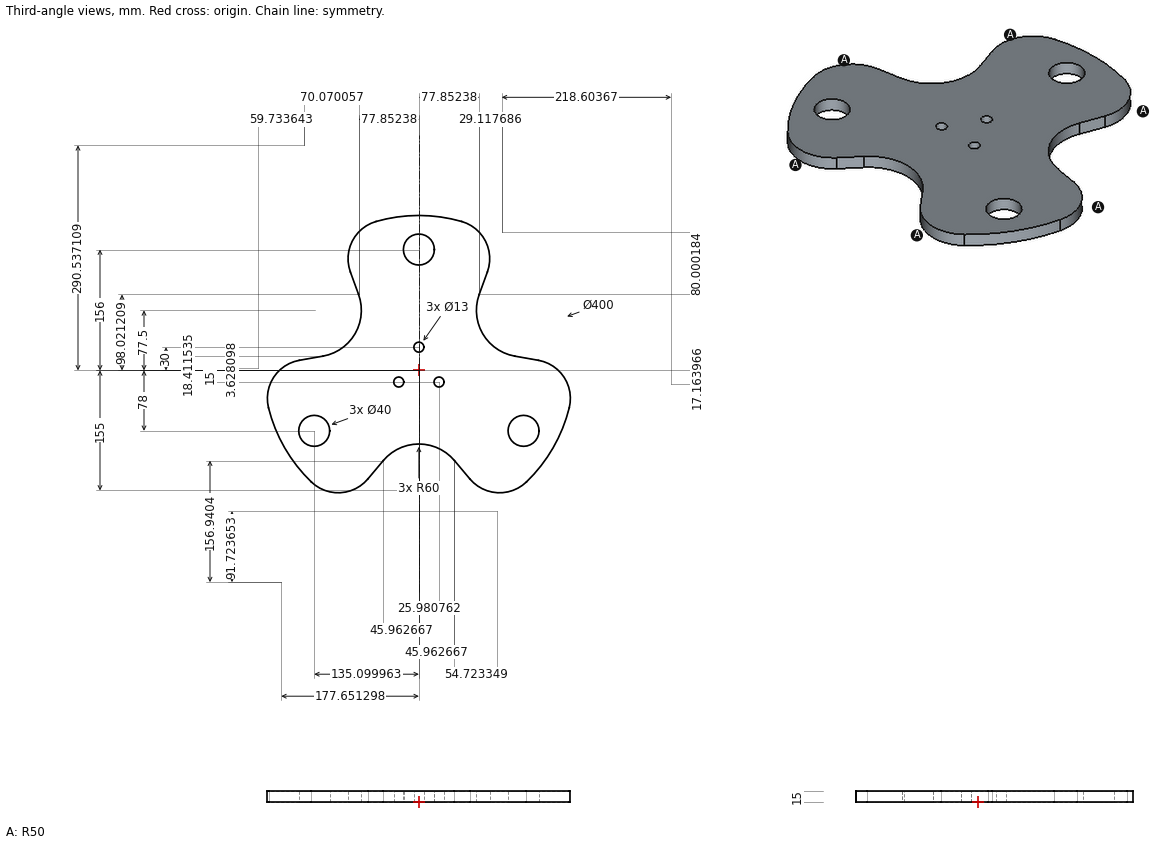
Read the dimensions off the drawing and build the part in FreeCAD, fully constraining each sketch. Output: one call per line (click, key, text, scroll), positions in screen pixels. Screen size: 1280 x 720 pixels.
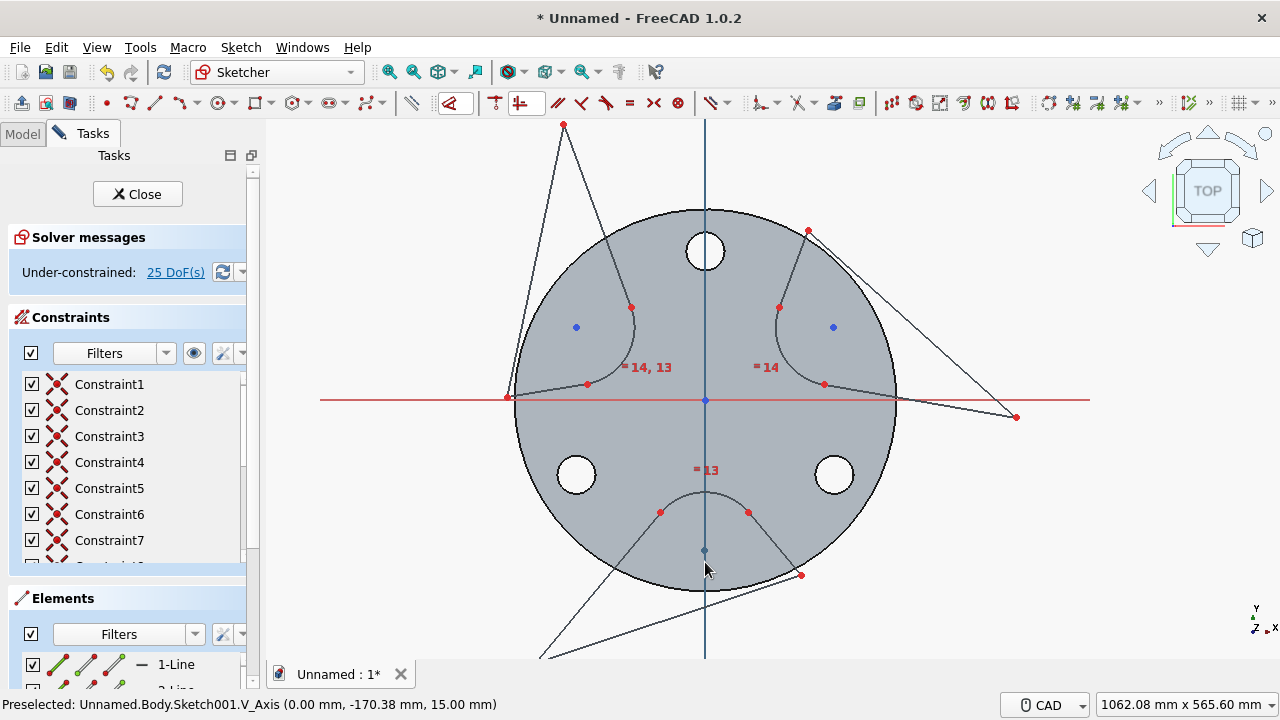
click(496, 104)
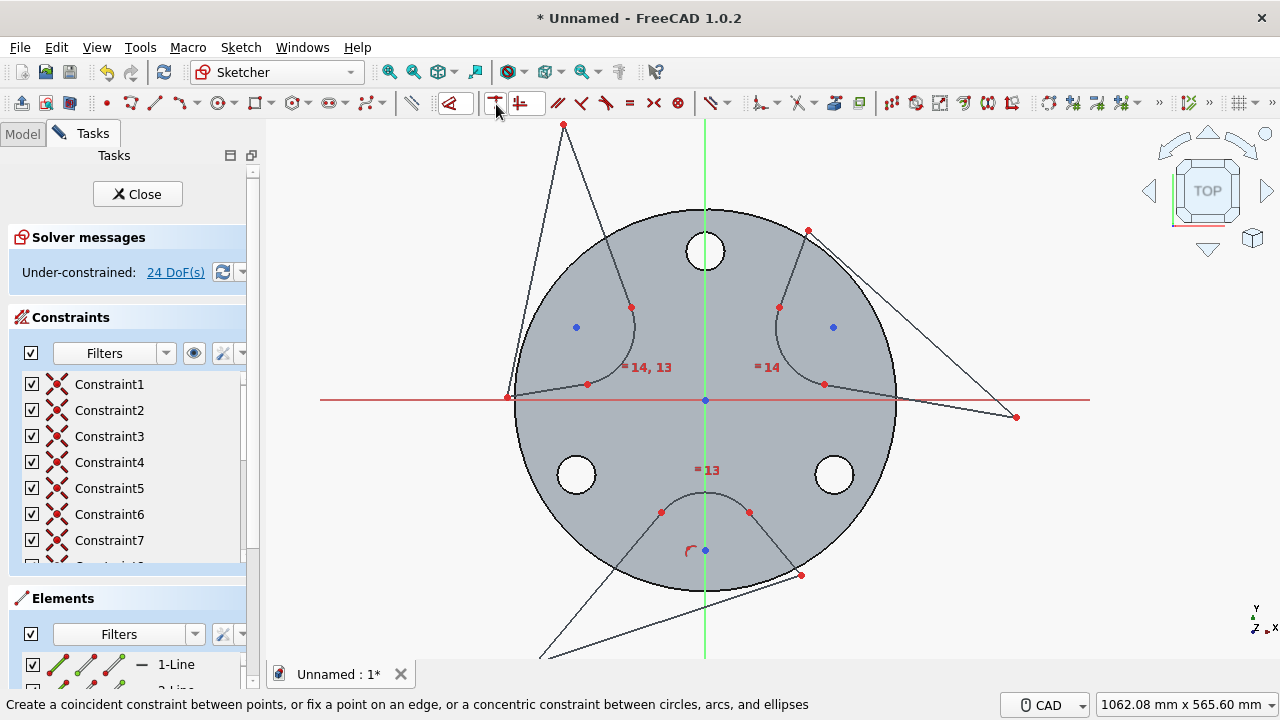
click(577, 327)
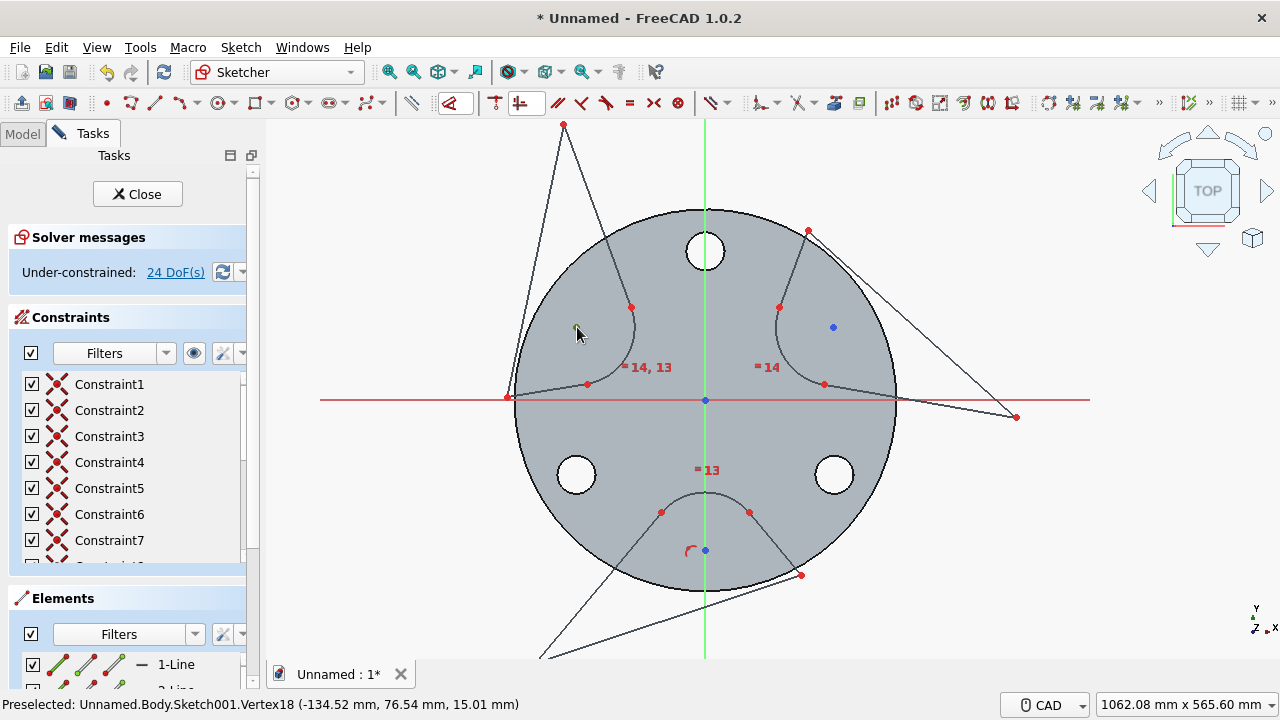
click(834, 328)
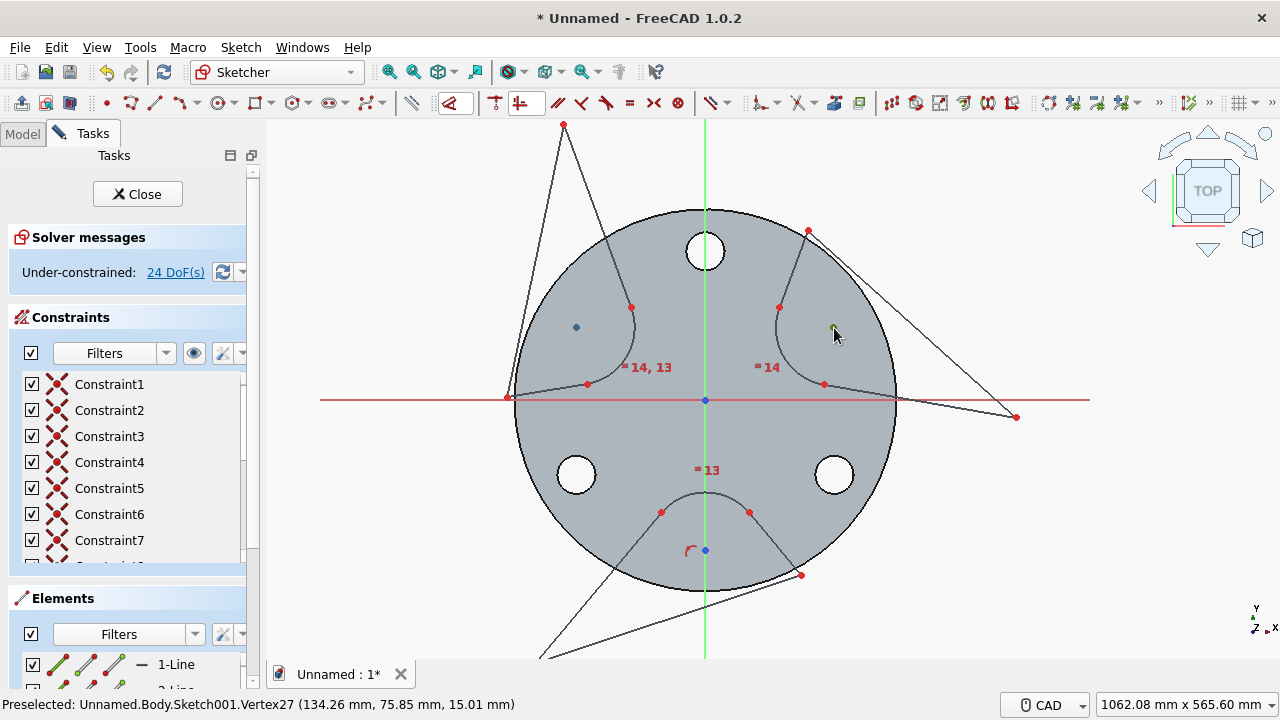
click(705, 562)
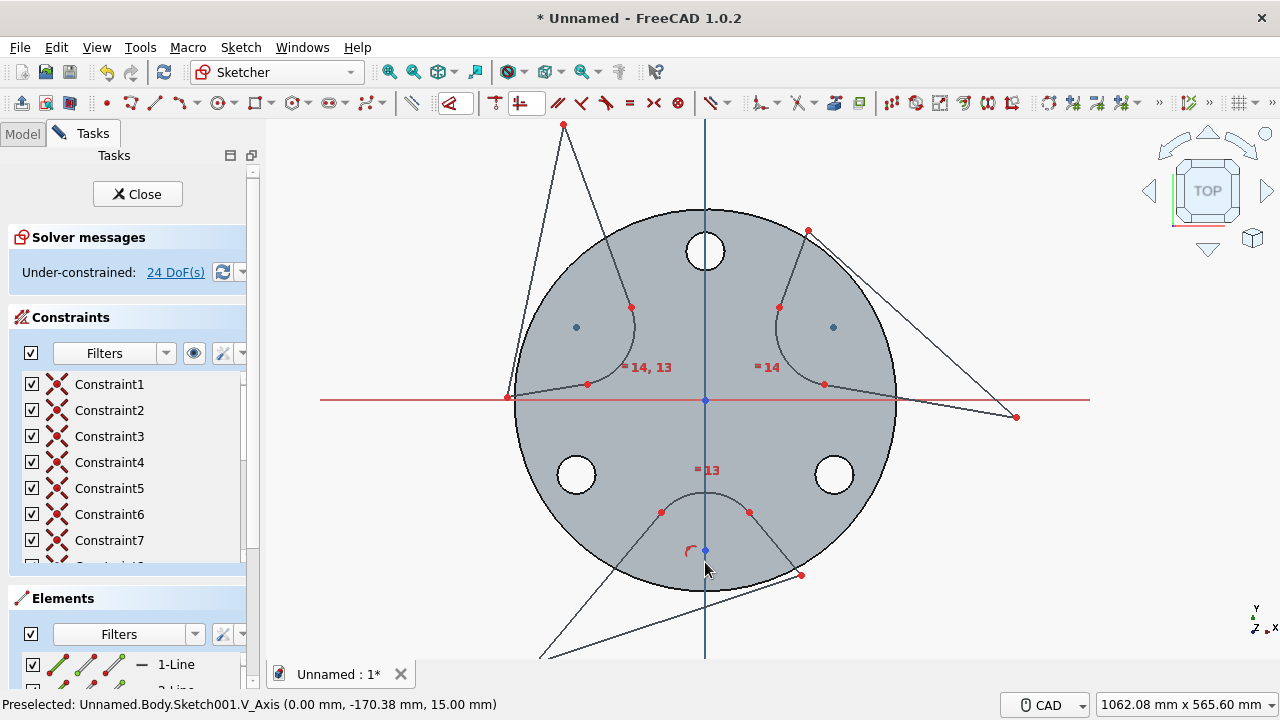
click(654, 104)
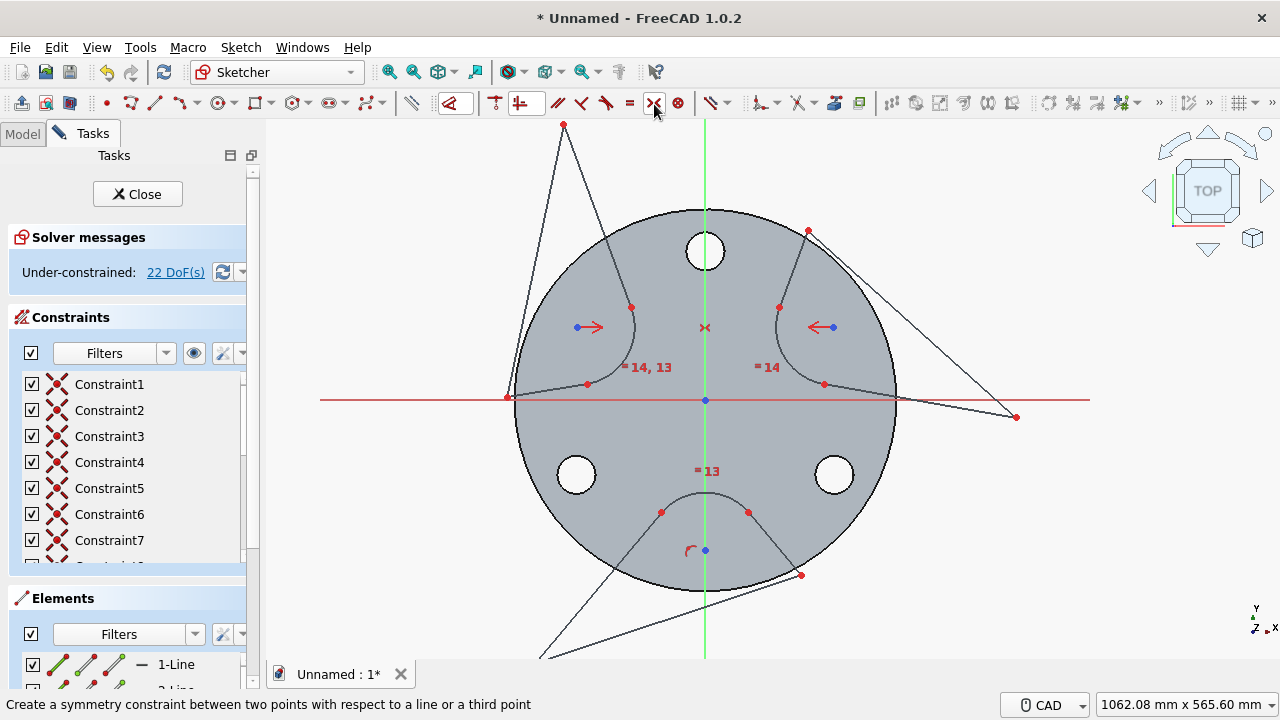
click(725, 496)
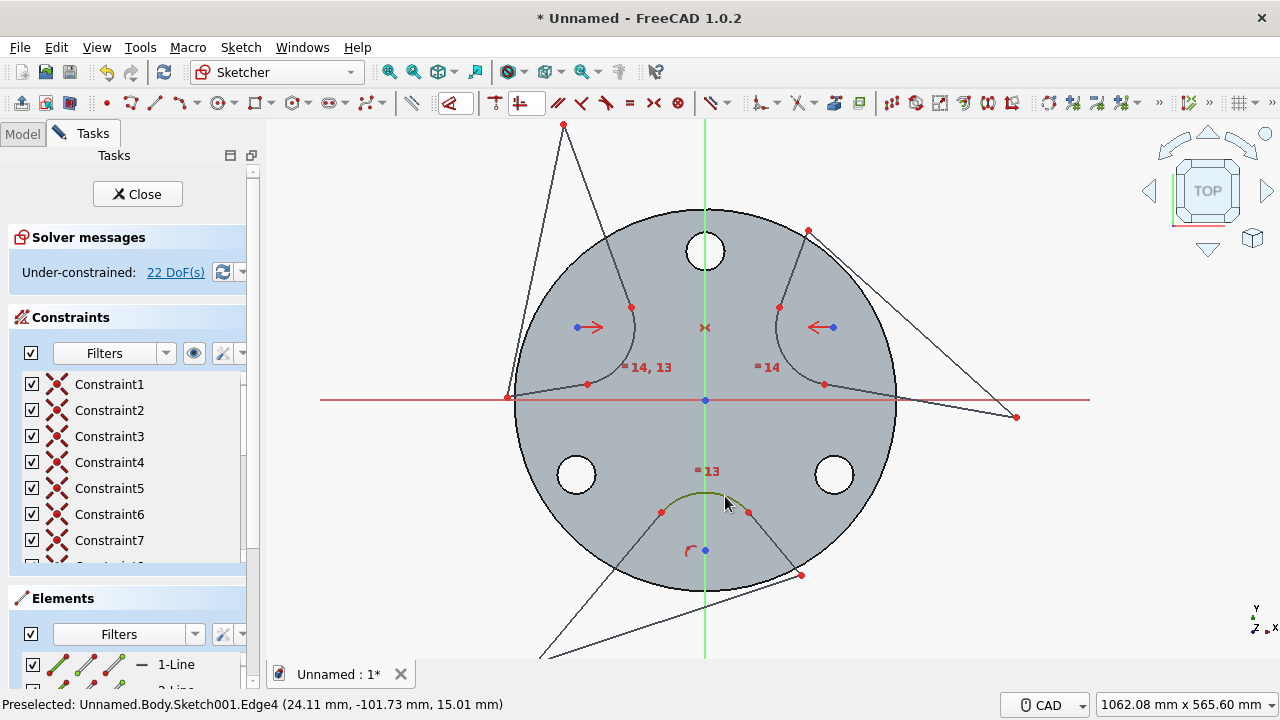
click(468, 104)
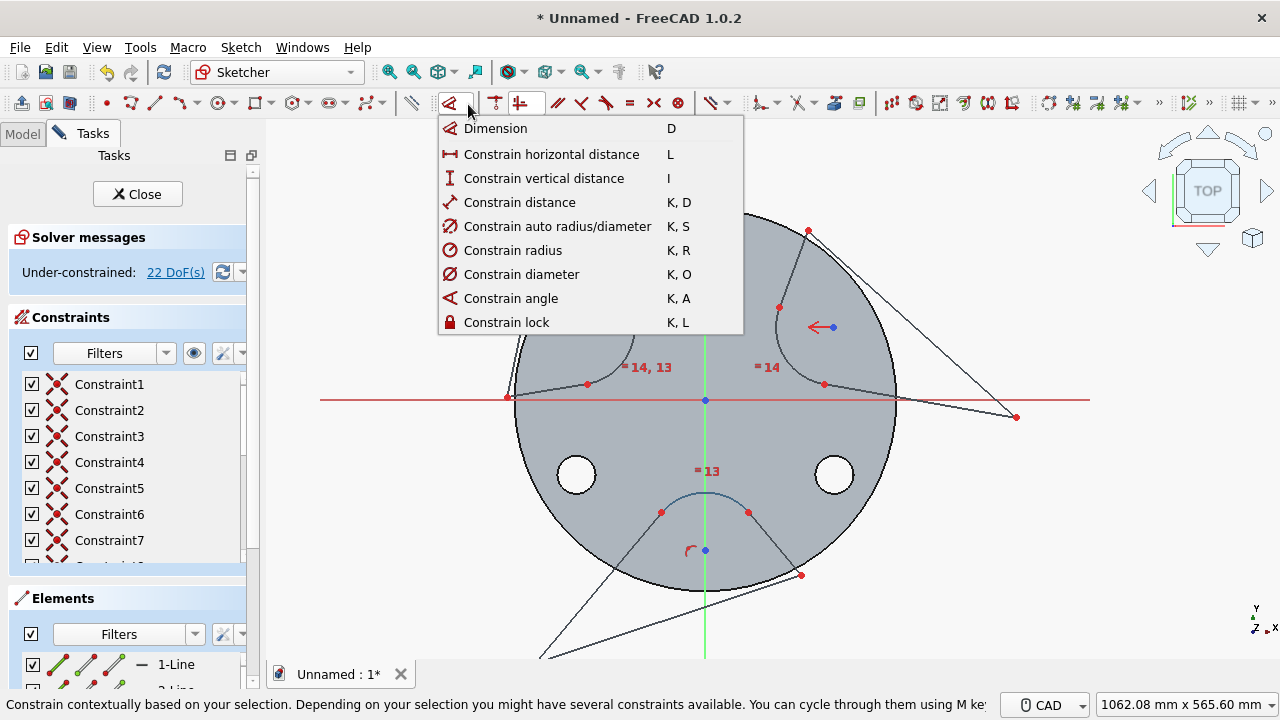
click(591, 250)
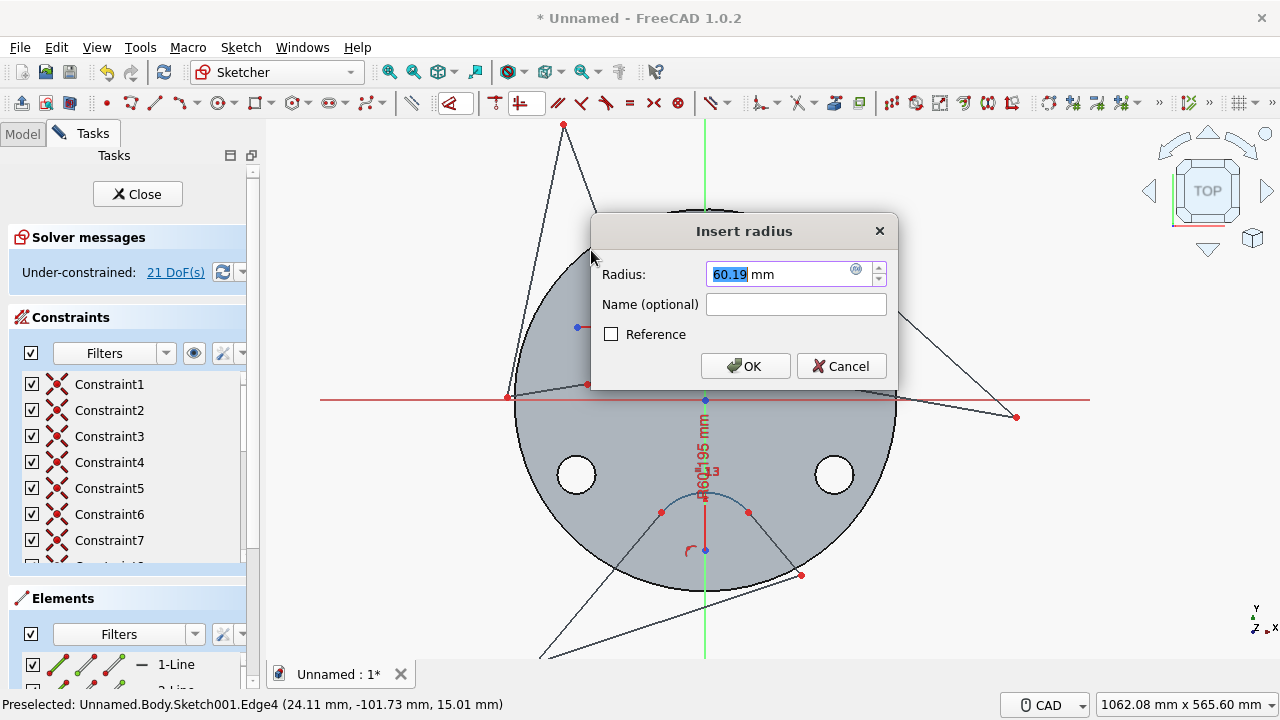
text(60)
key(Return)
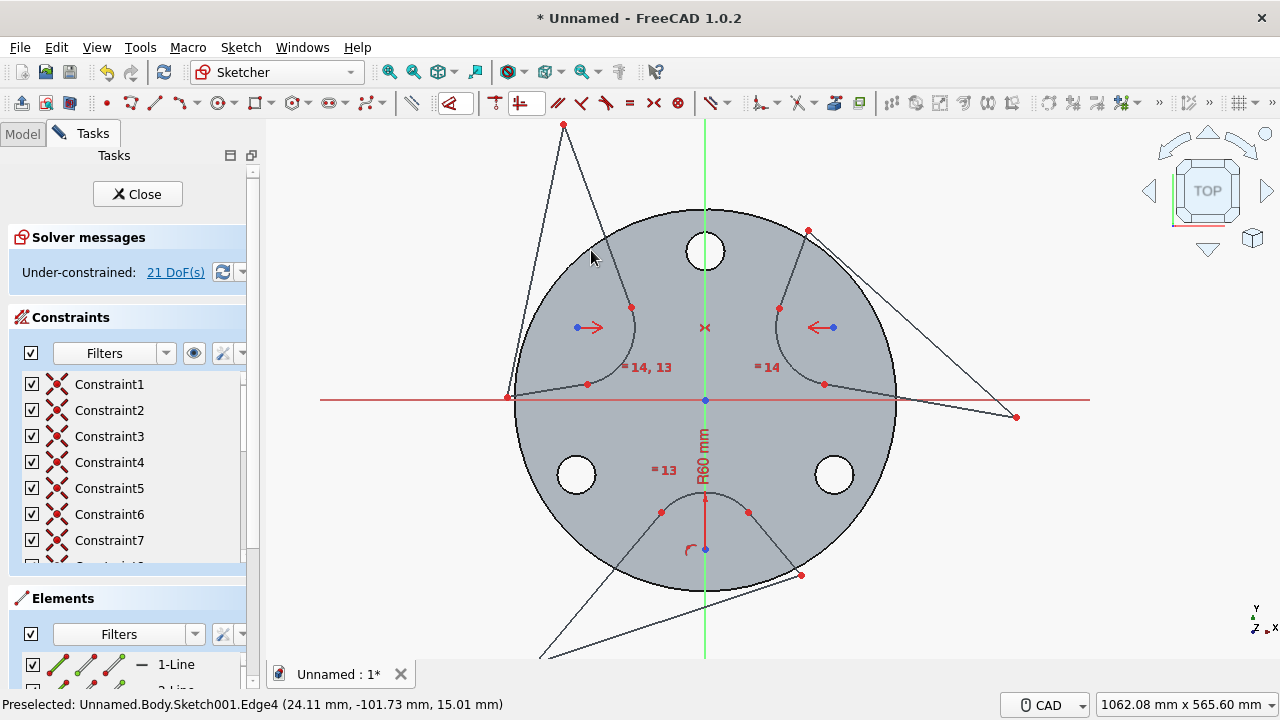
click(705, 550)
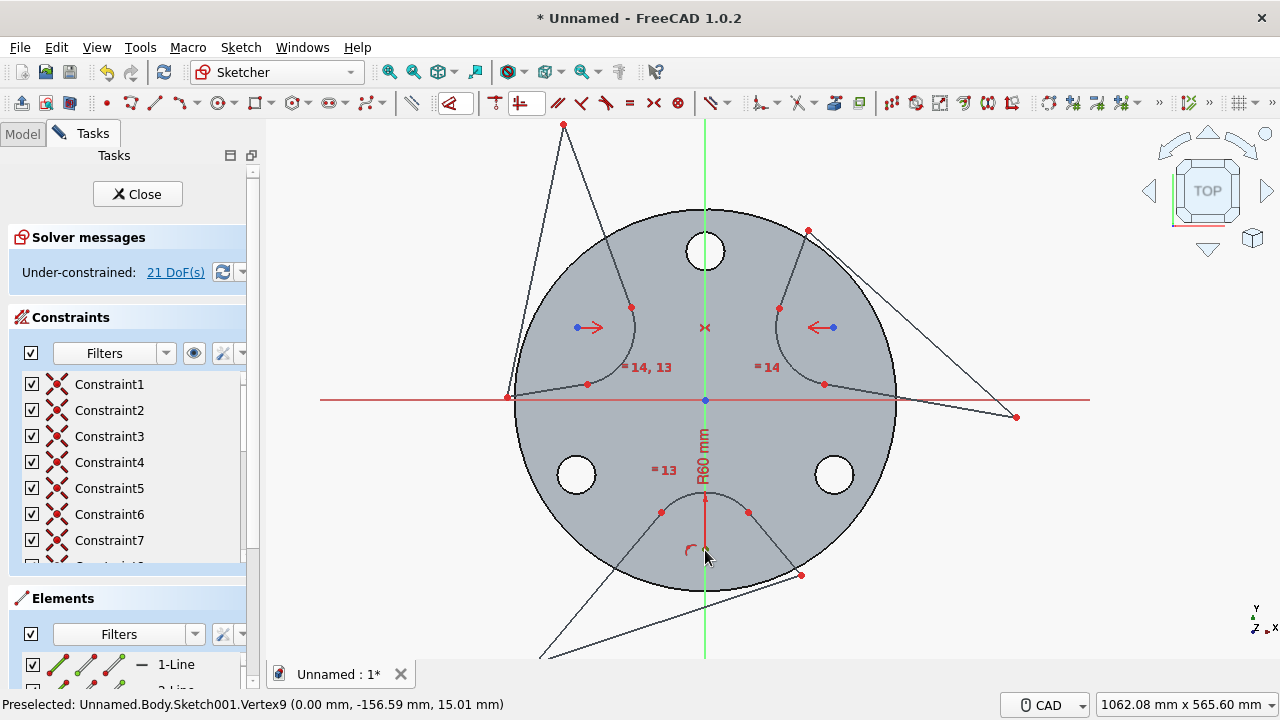
click(468, 104)